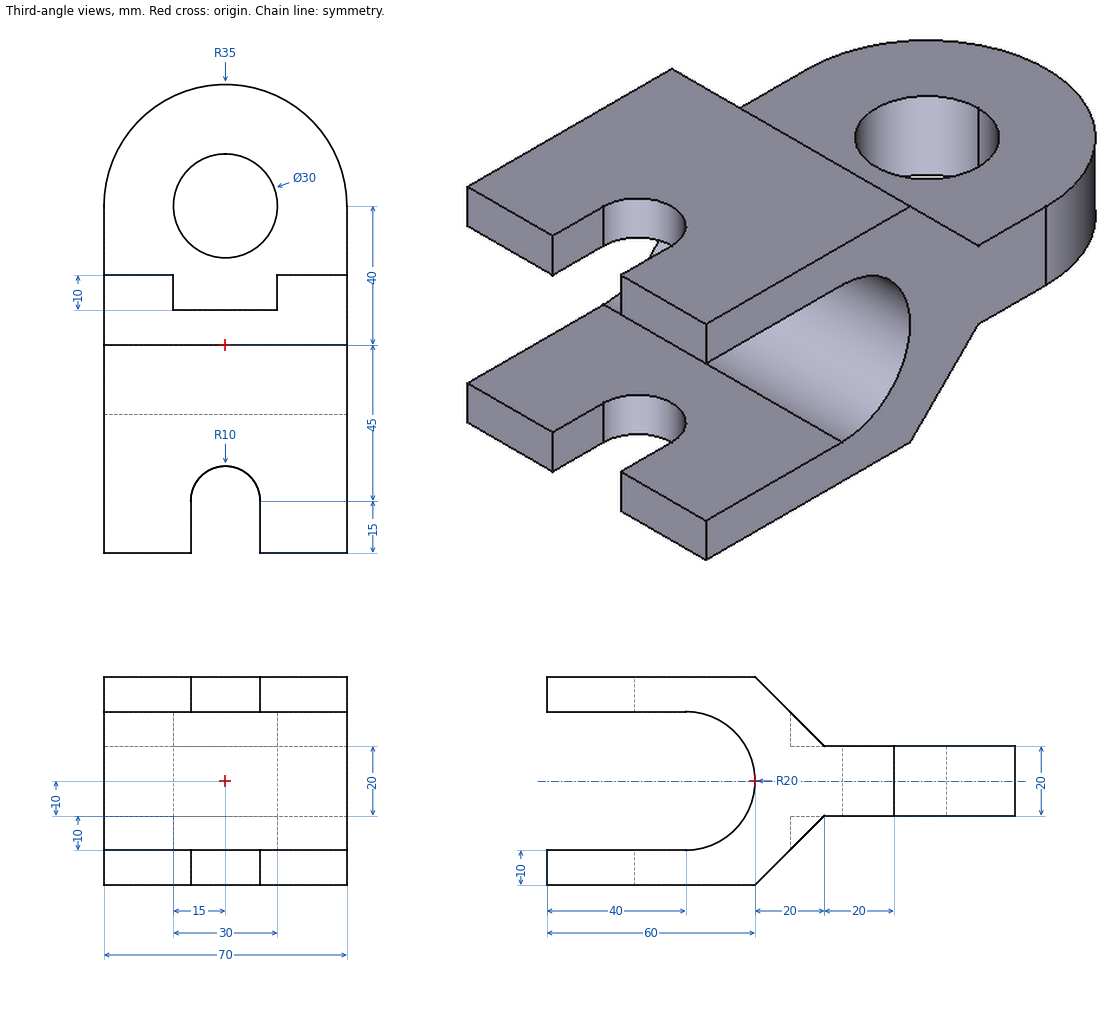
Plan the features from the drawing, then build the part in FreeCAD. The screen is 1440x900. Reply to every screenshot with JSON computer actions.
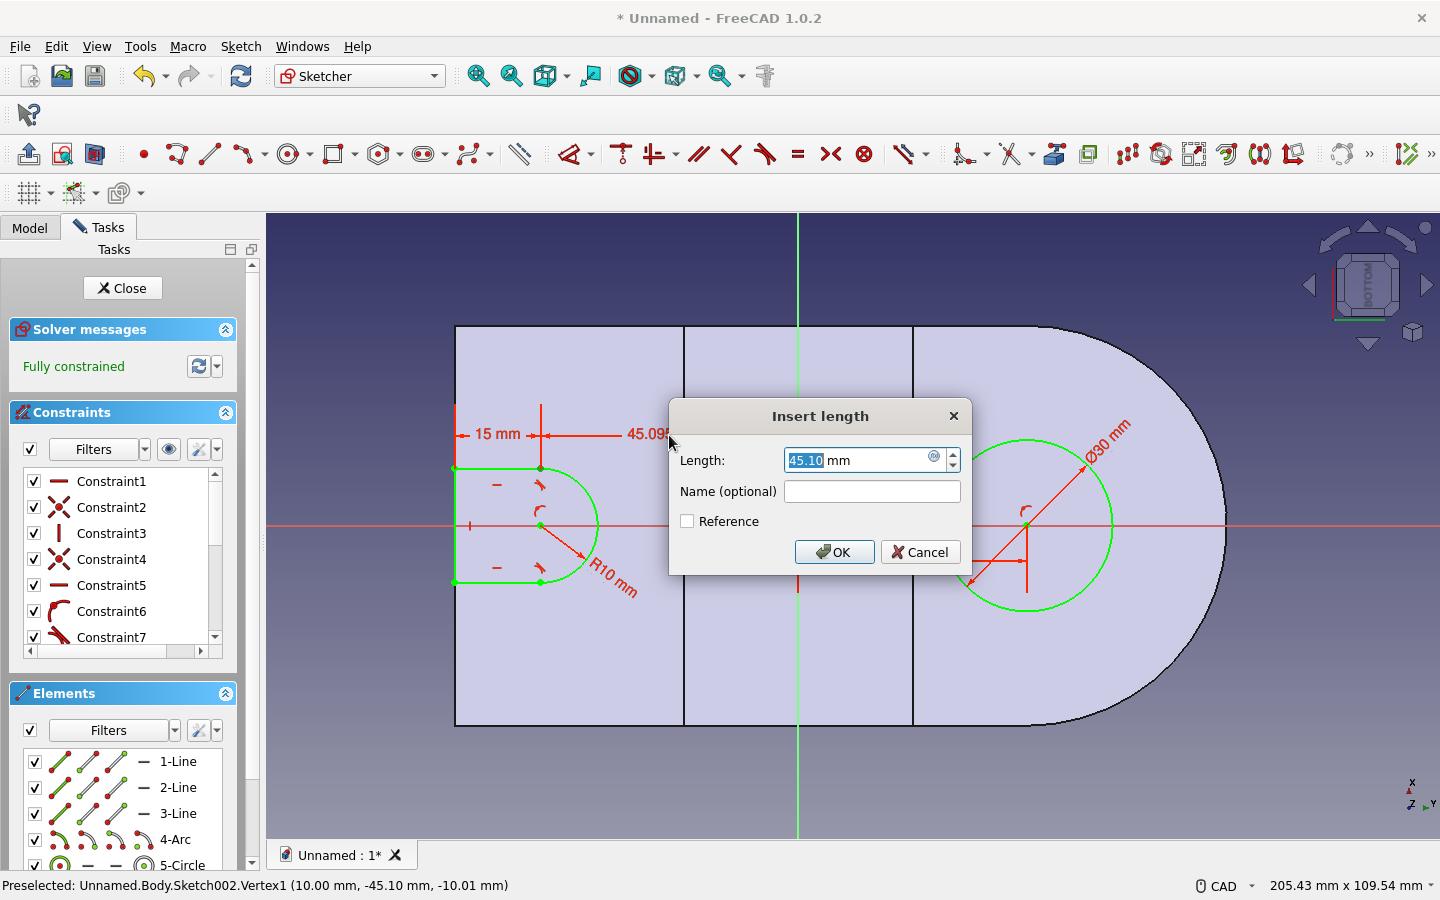
{"action": "type", "text": "45"}
{"action": "key", "text": "Return"}
{"action": "key", "text": "Escape"}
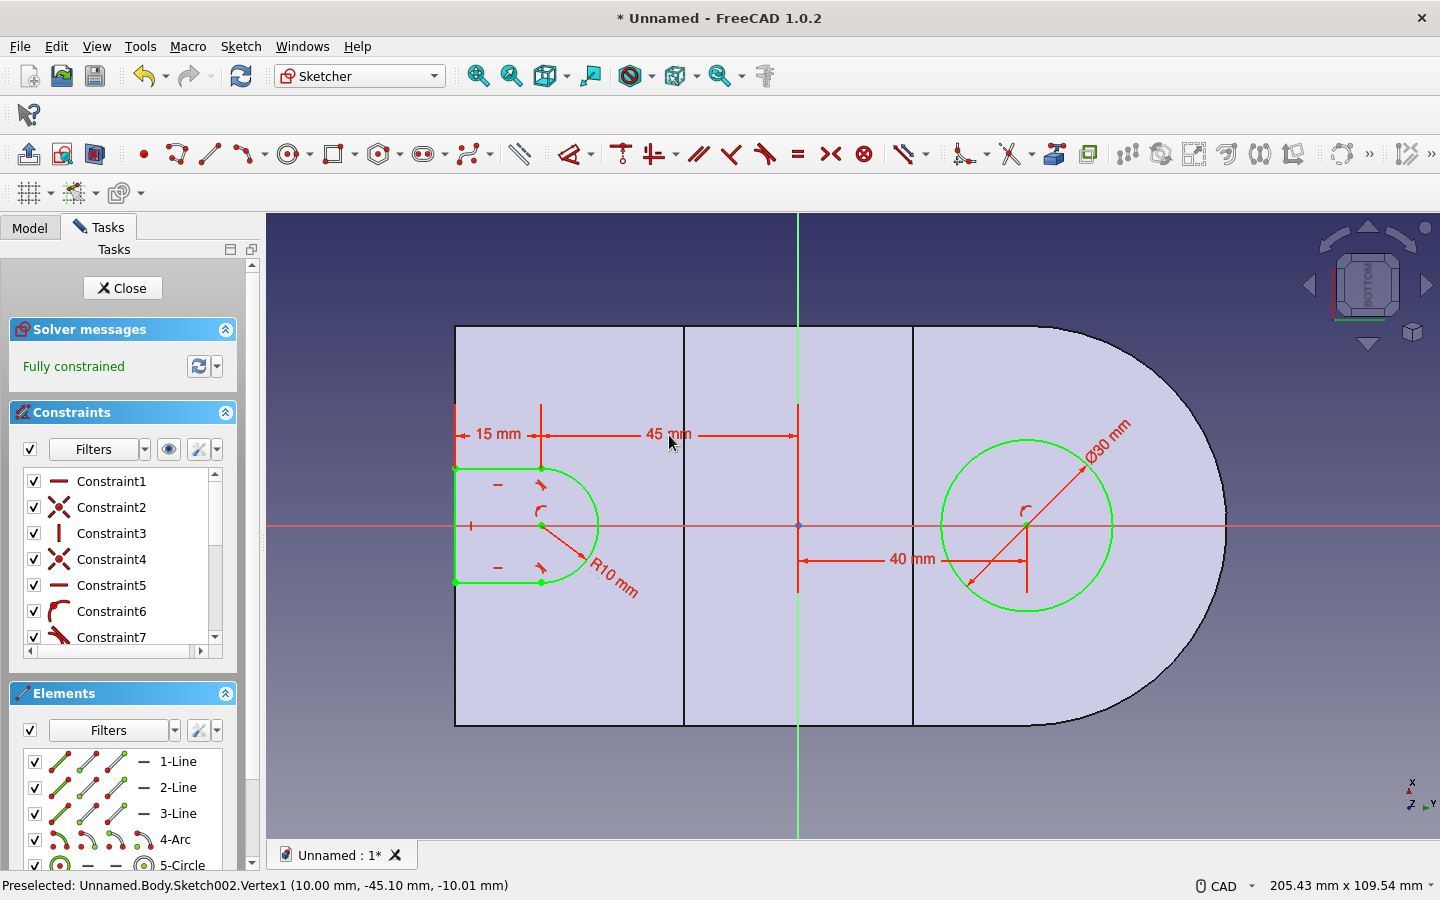
{"action": "left_click", "coordinate": [123, 288]}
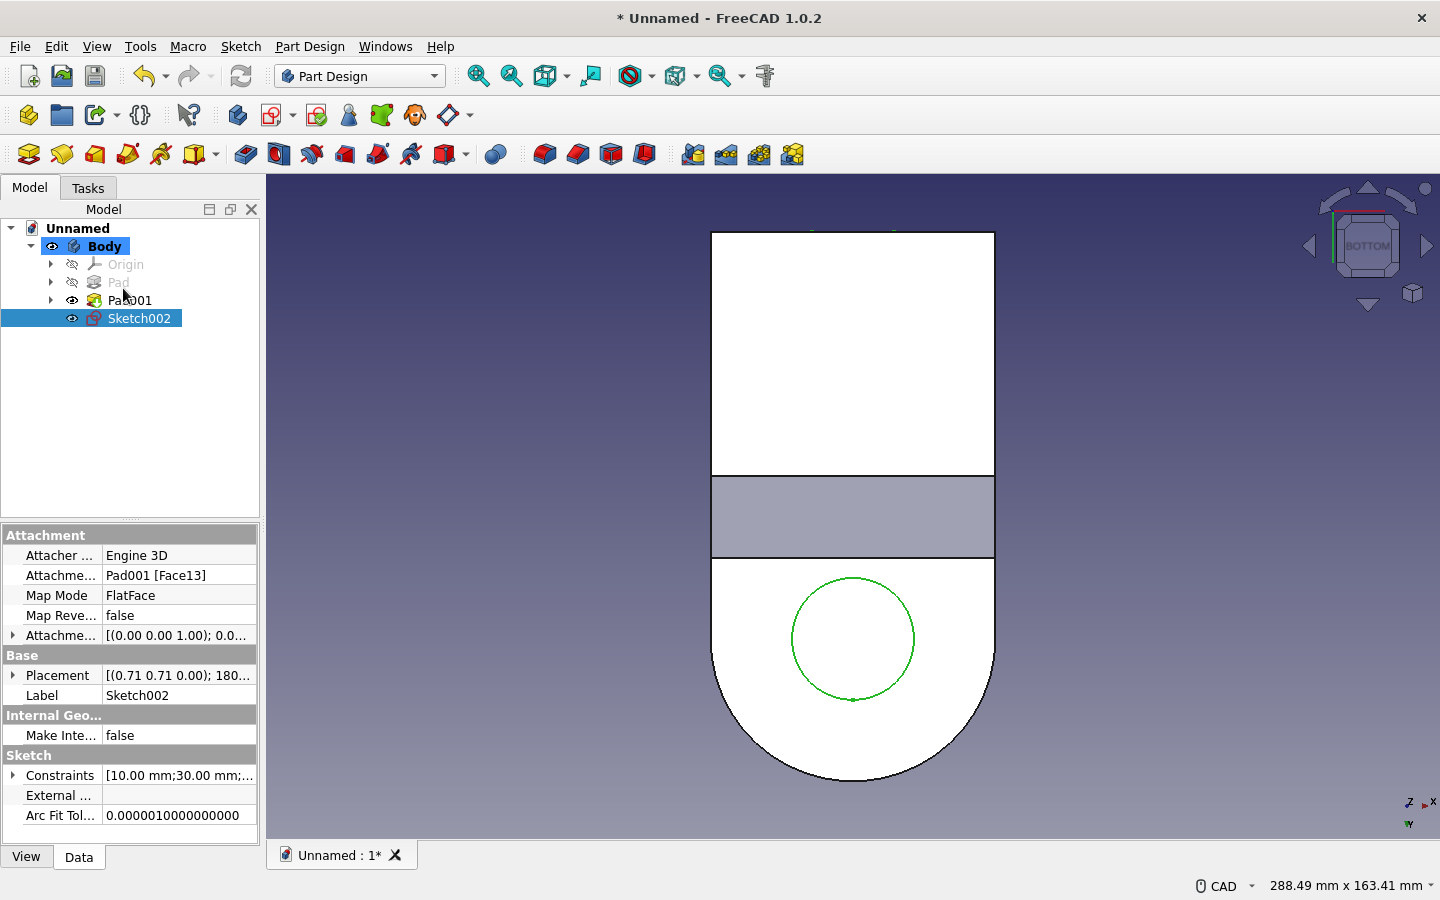
{"action": "left_click", "coordinate": [246, 154]}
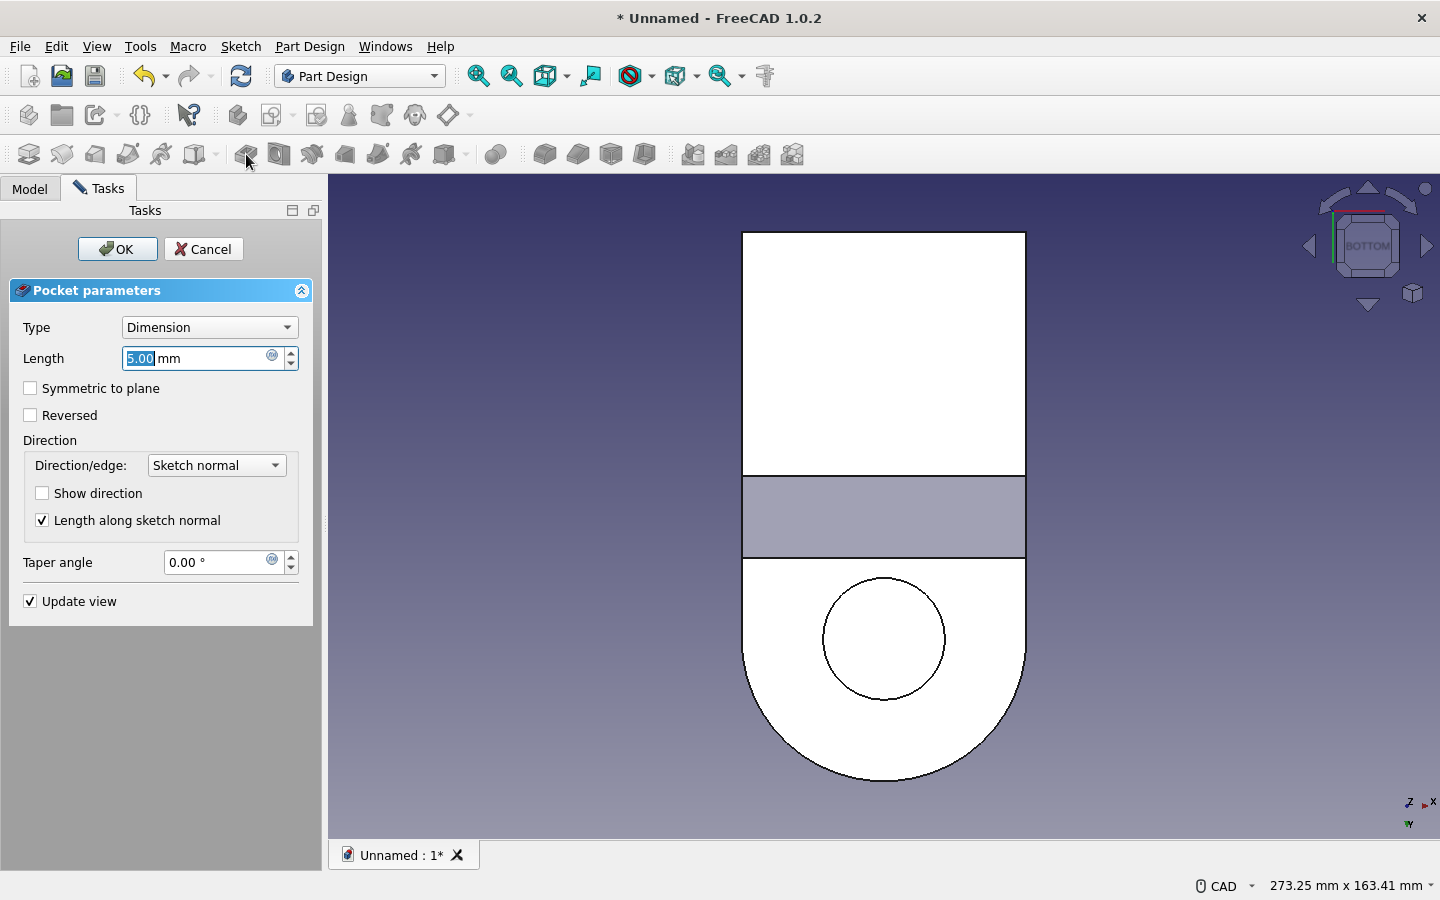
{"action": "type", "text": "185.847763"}
{"action": "key", "text": "Tab"}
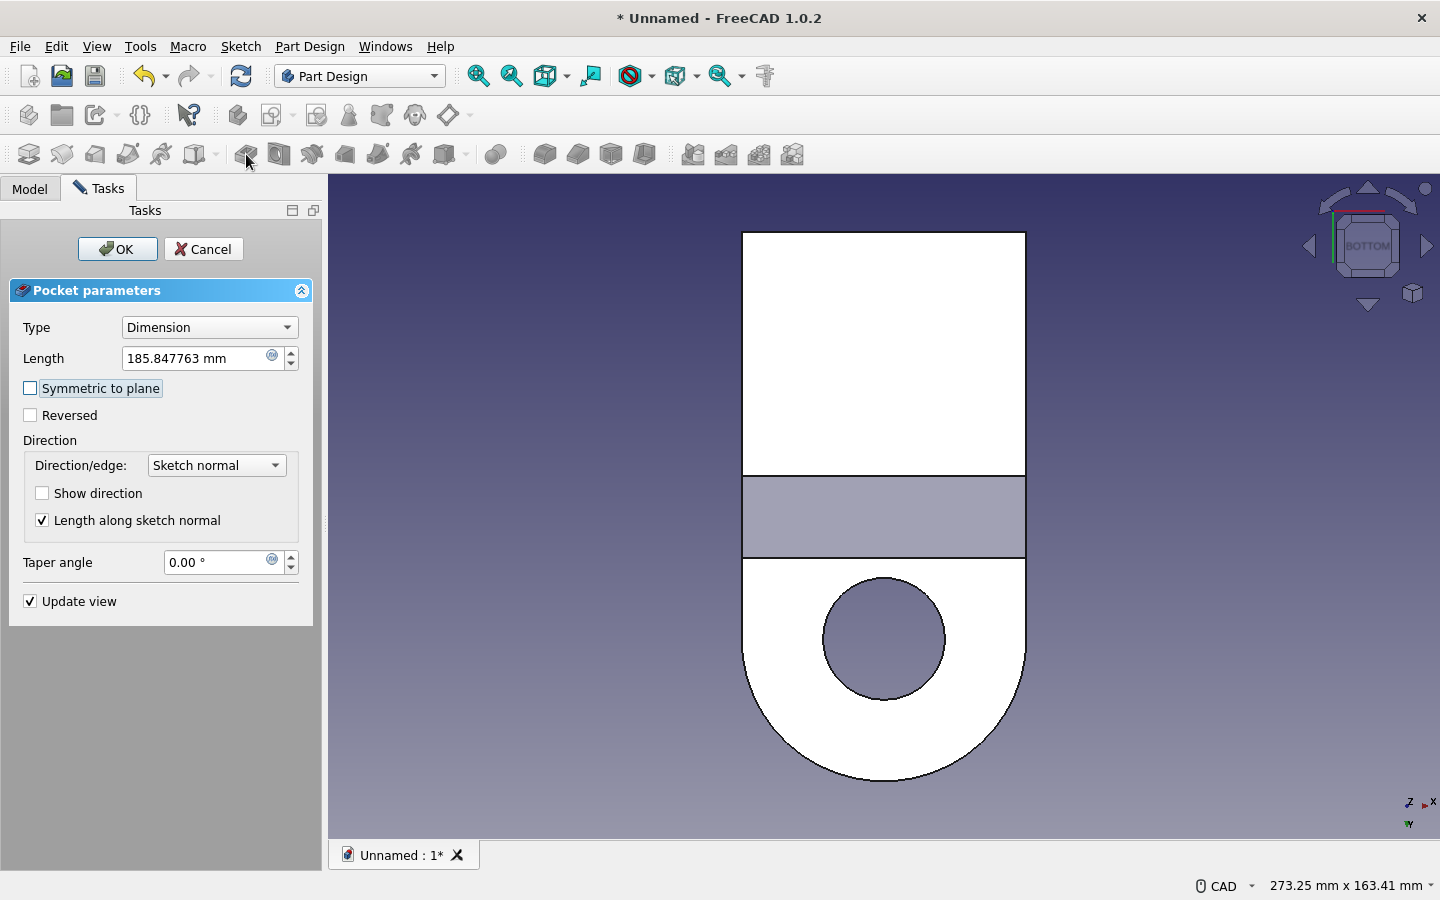
{"action": "left_click", "coordinate": [31, 388]}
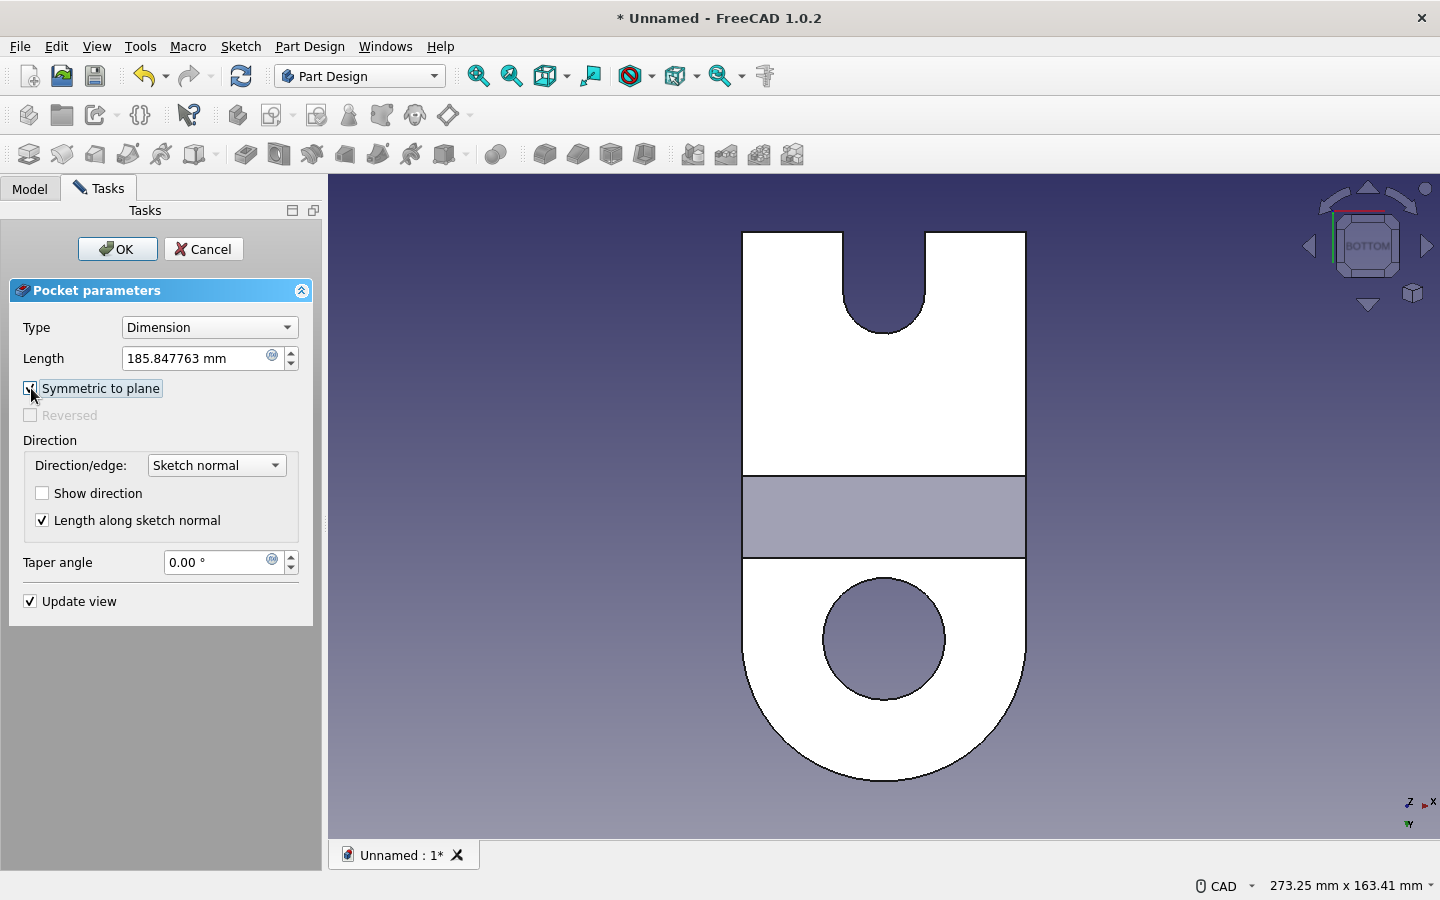
{"action": "left_click", "coordinate": [118, 249]}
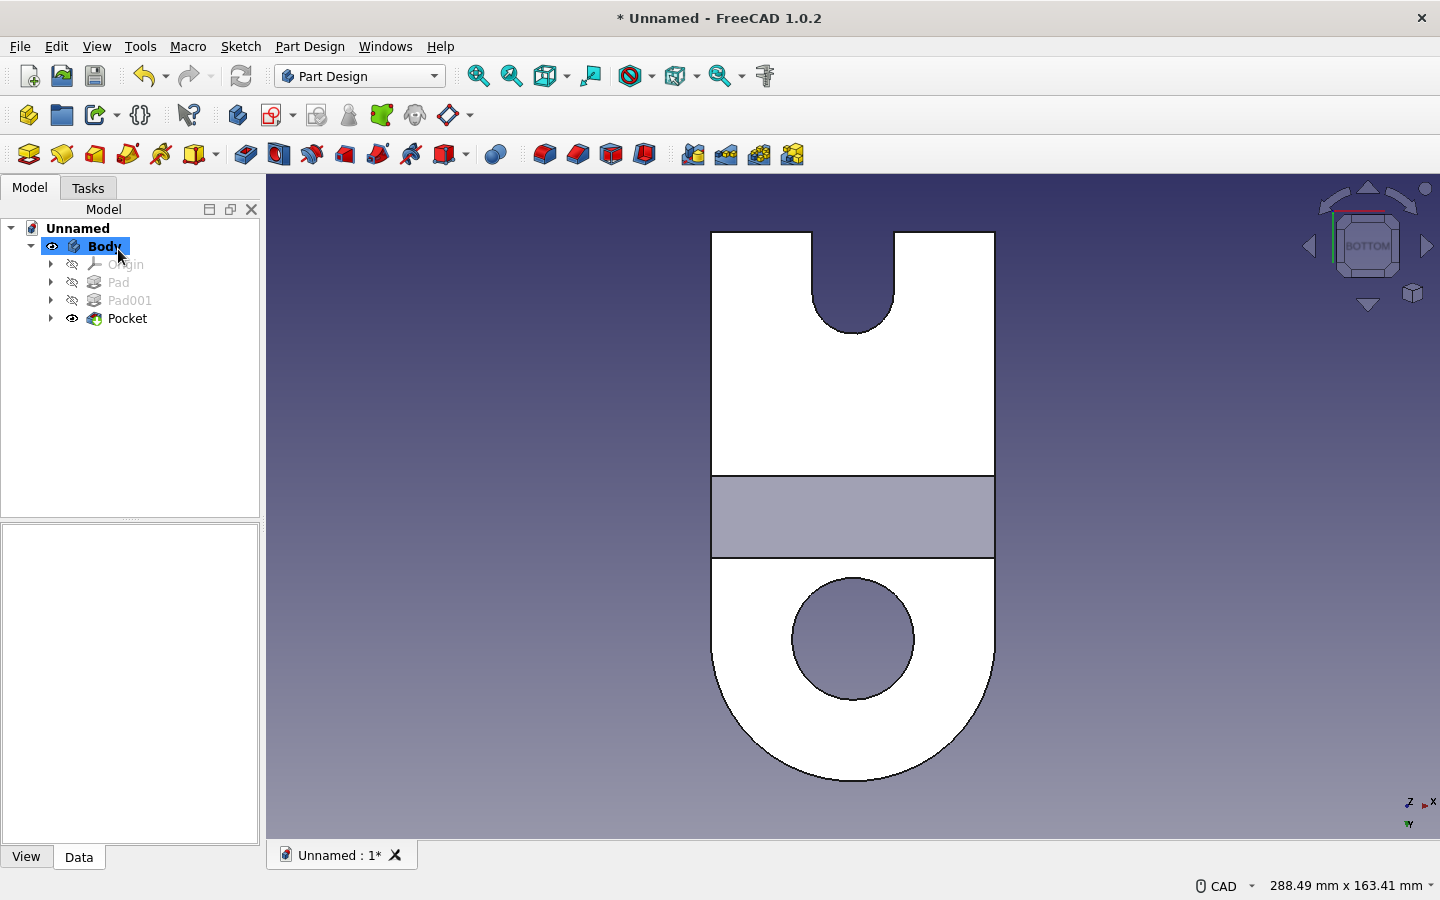
{"action": "left_click", "coordinate": [51, 264]}